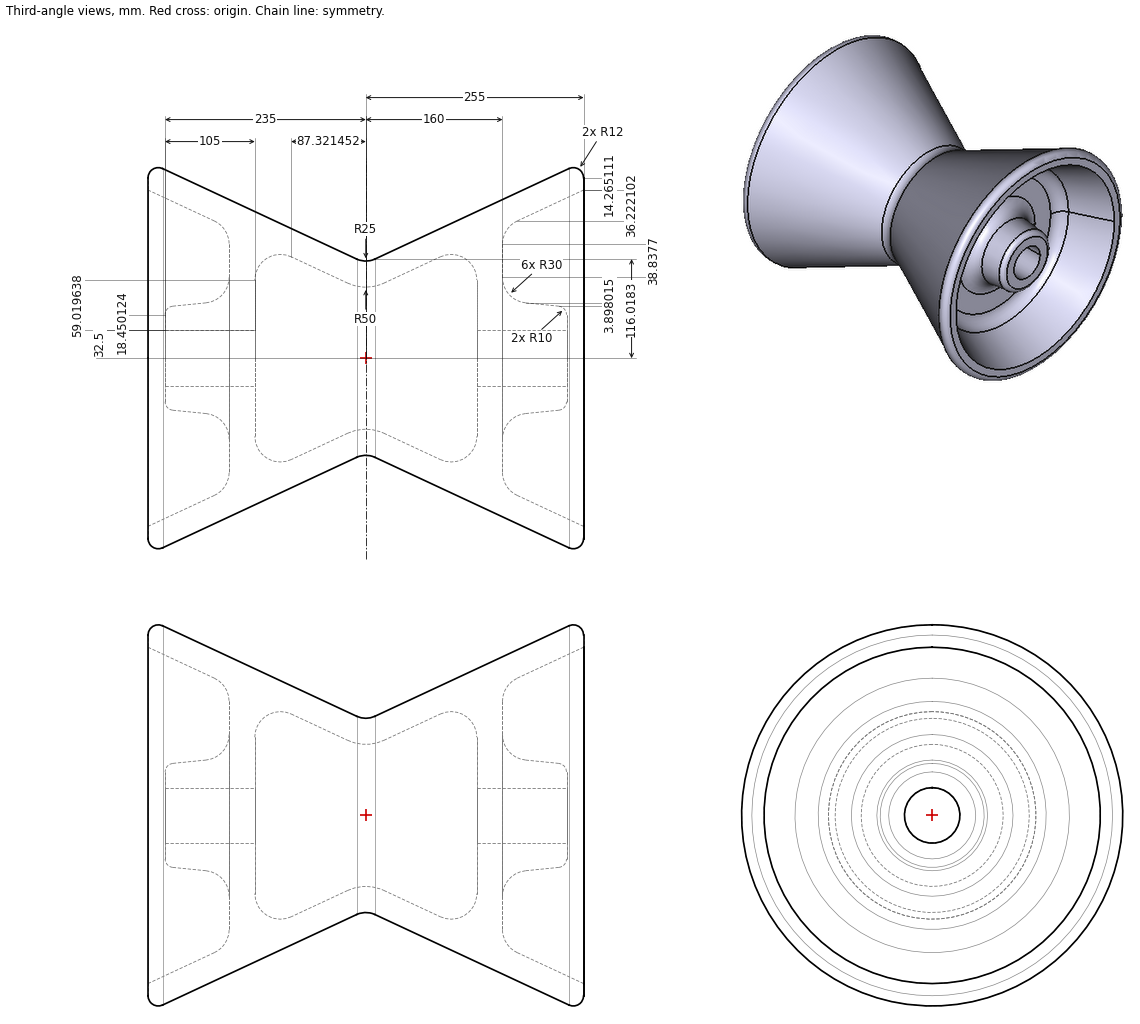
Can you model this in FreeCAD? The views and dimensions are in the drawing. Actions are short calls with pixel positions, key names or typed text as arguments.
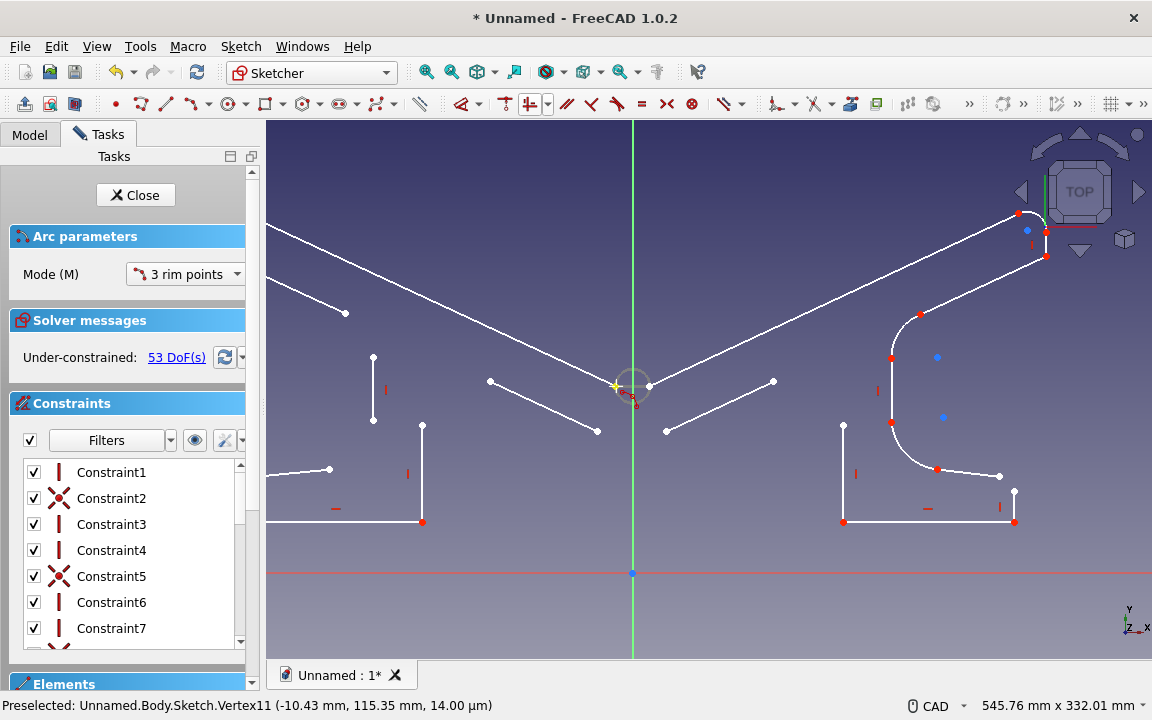
scroll(629, 389, up, 8)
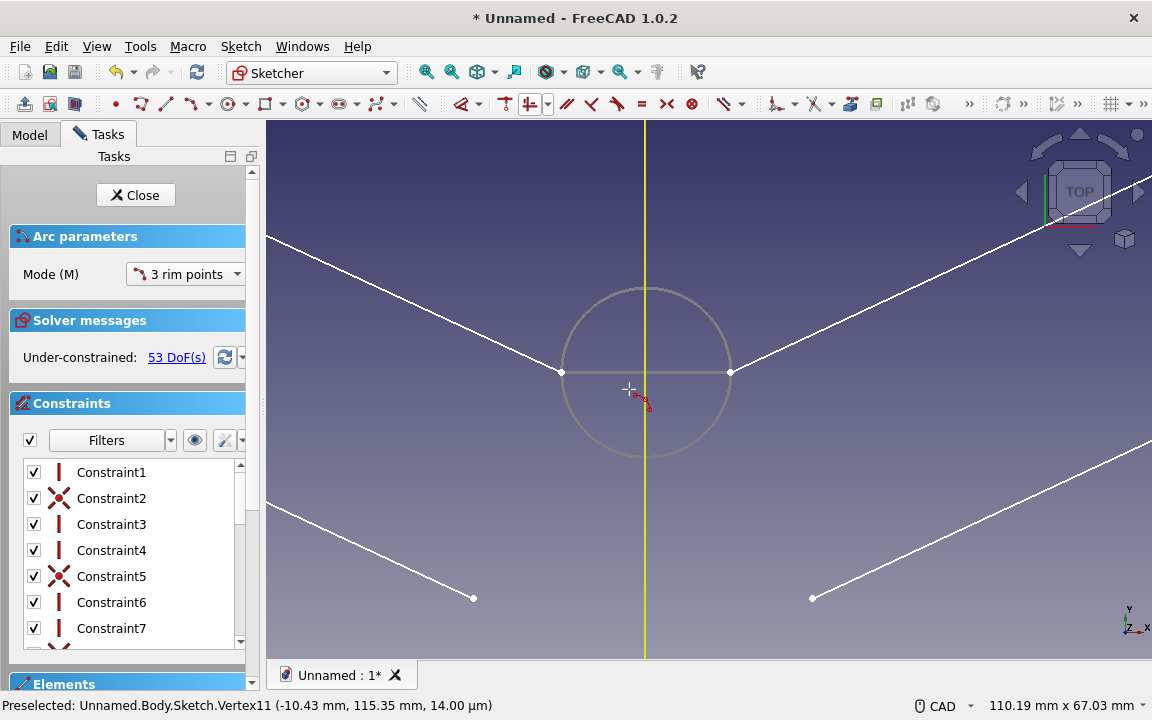
click(628, 385)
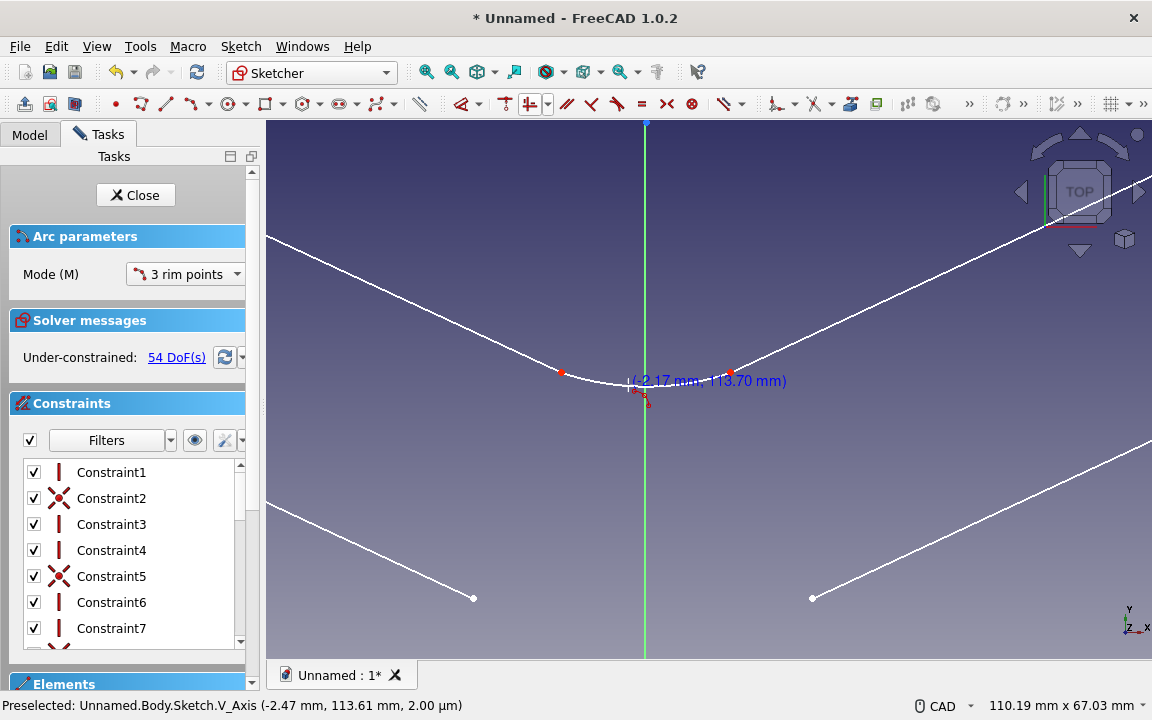
scroll(640, 387, down, 11)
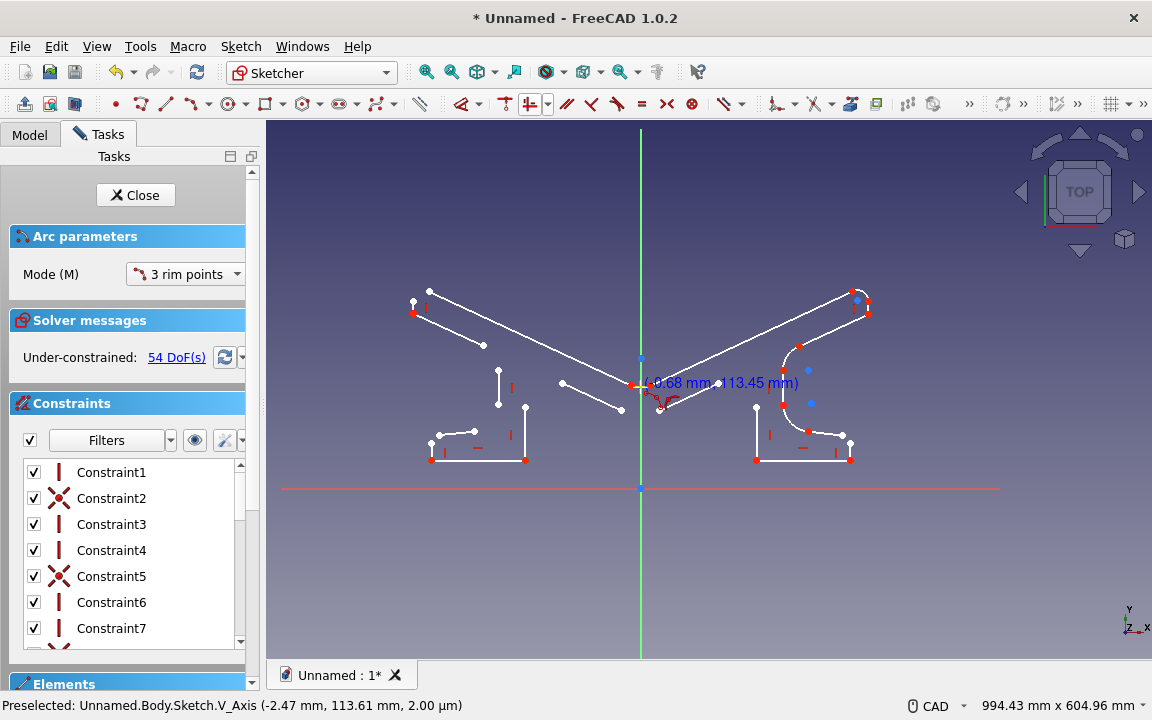
click(429, 292)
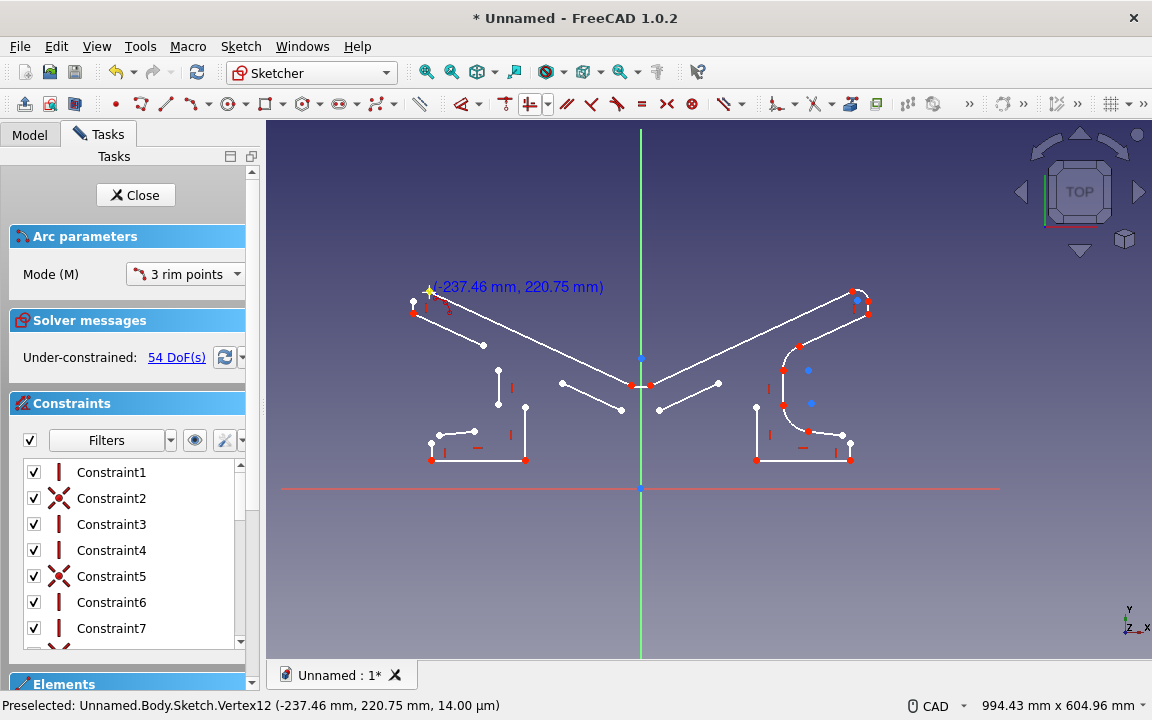
scroll(414, 300, up, 5)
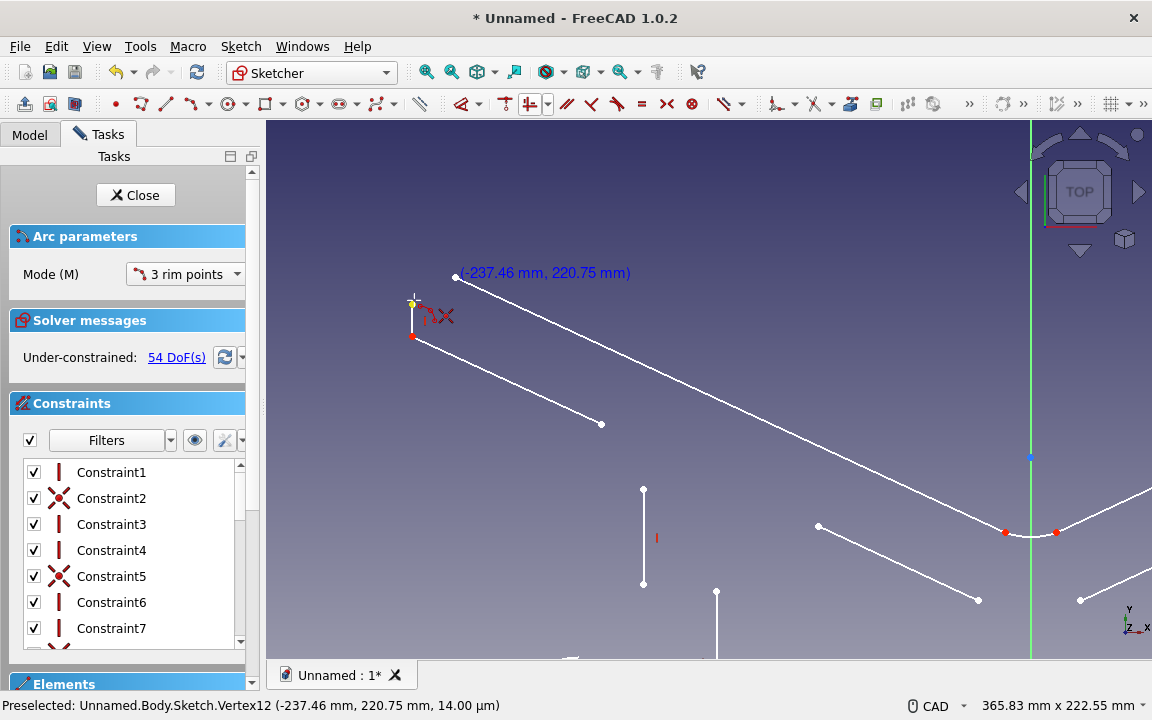
click(412, 305)
click(427, 276)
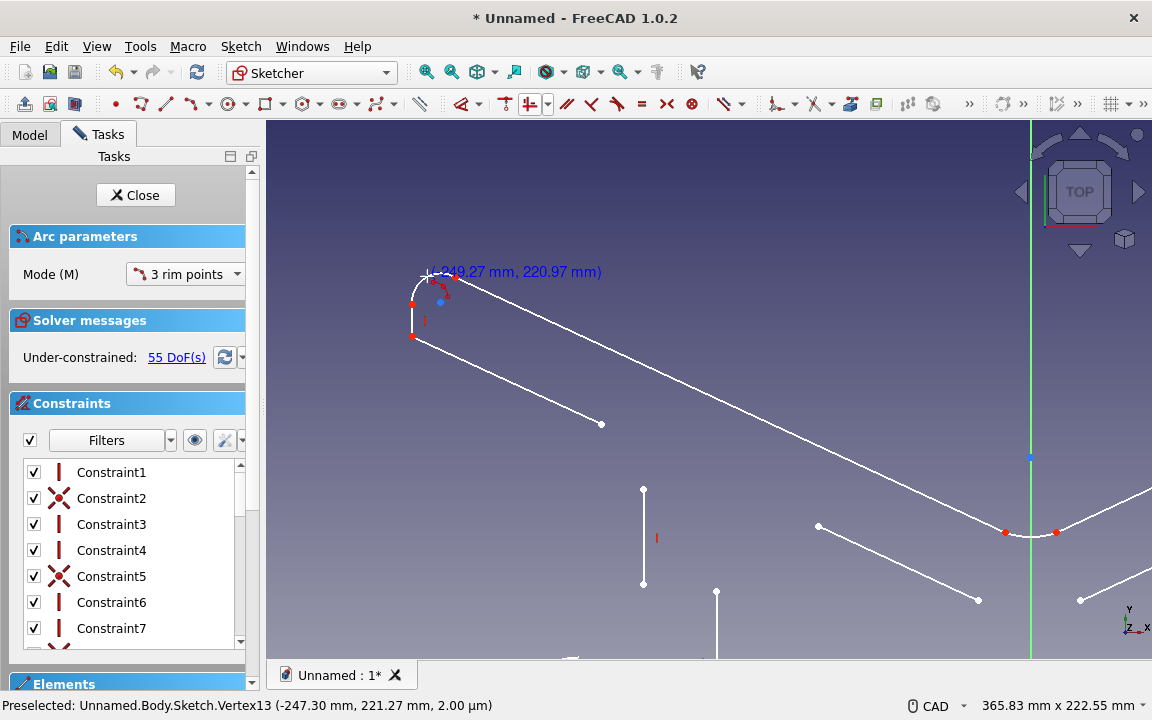
click(602, 424)
click(644, 490)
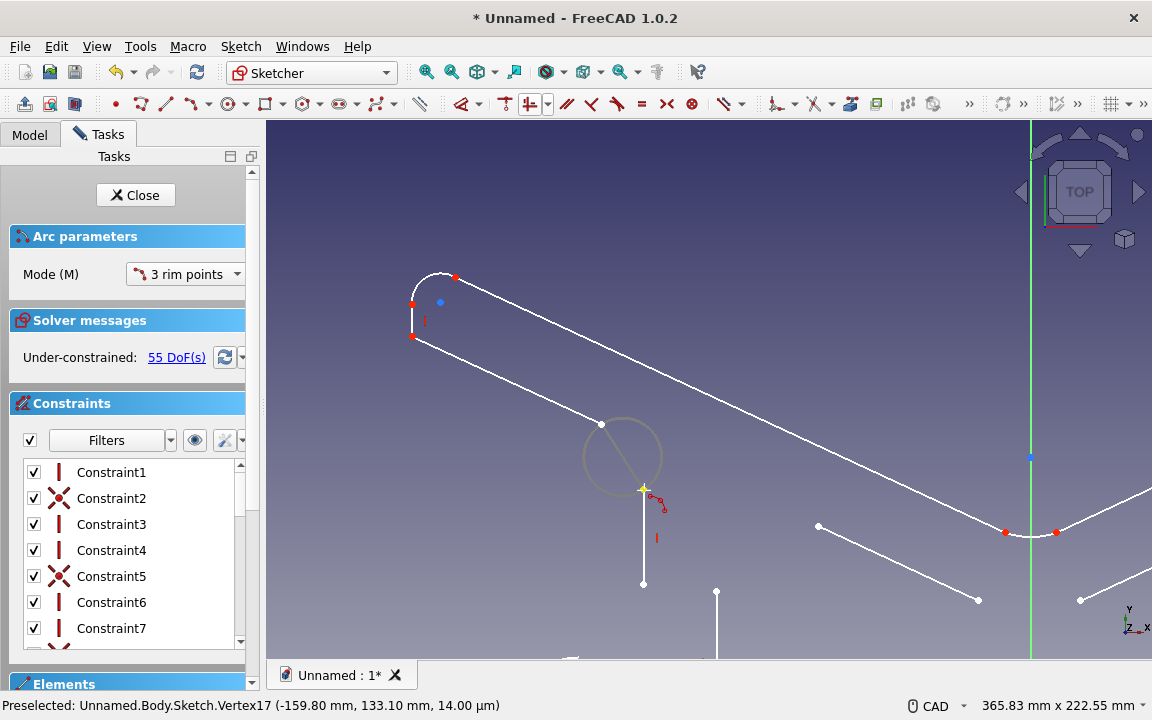
scroll(632, 450, up, 2)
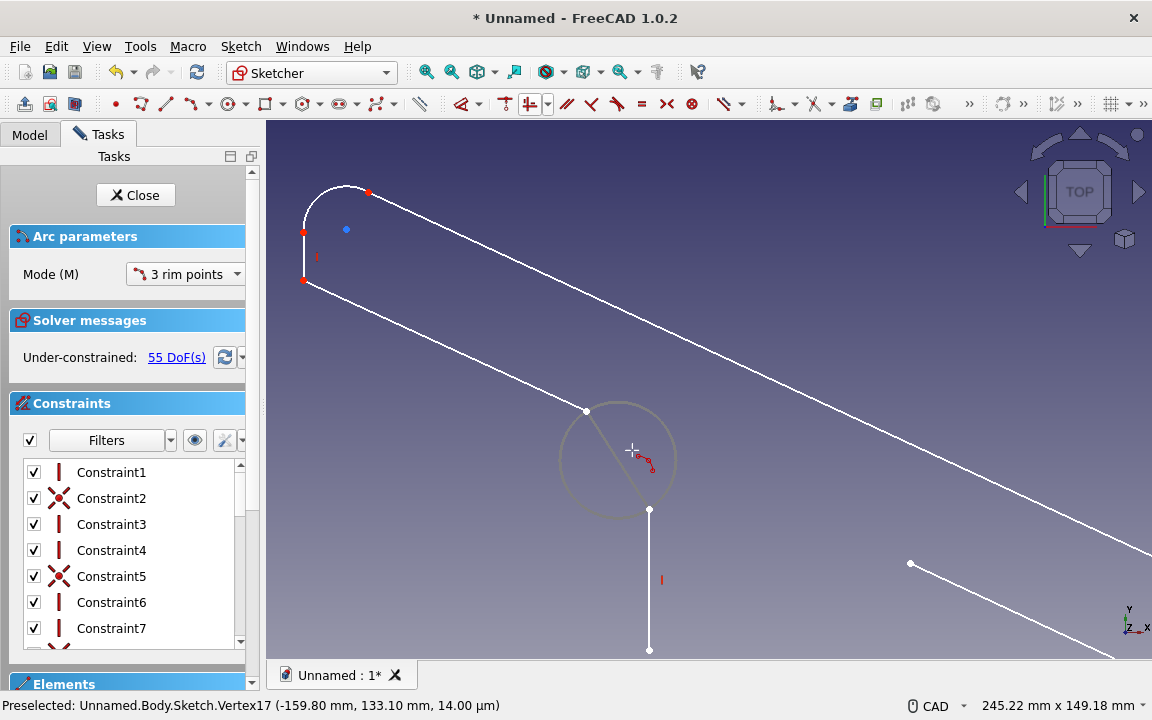
click(632, 449)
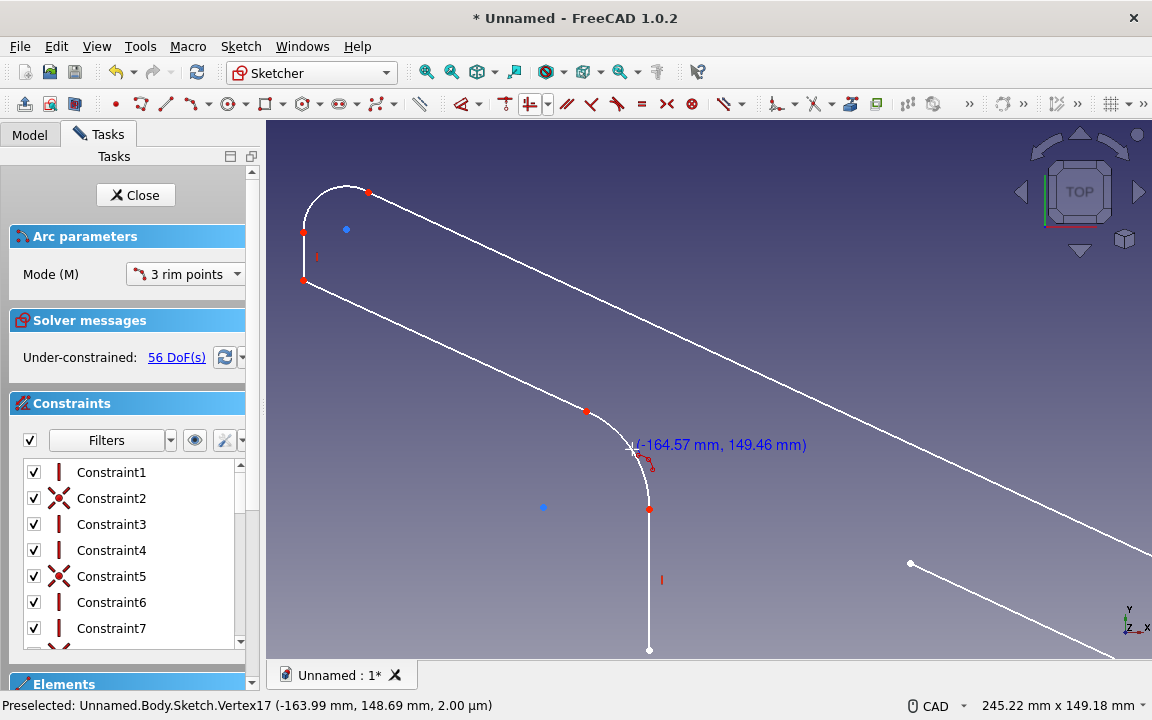
scroll(449, 324, down, 7)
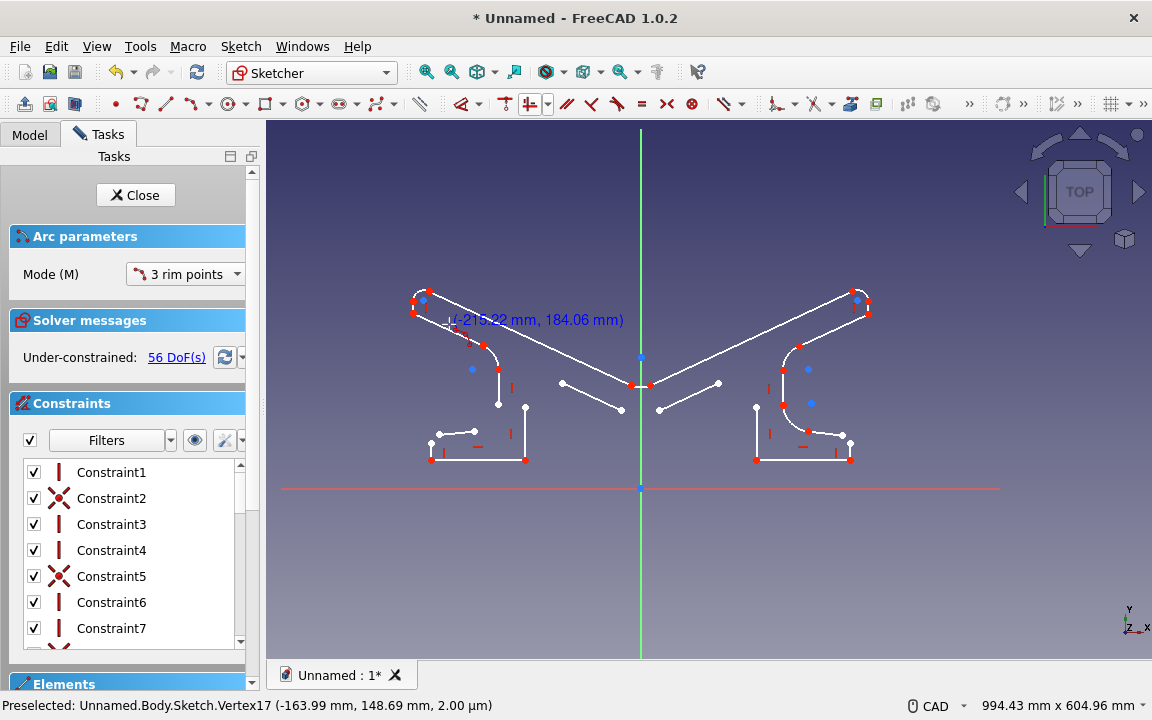
click(499, 405)
click(474, 432)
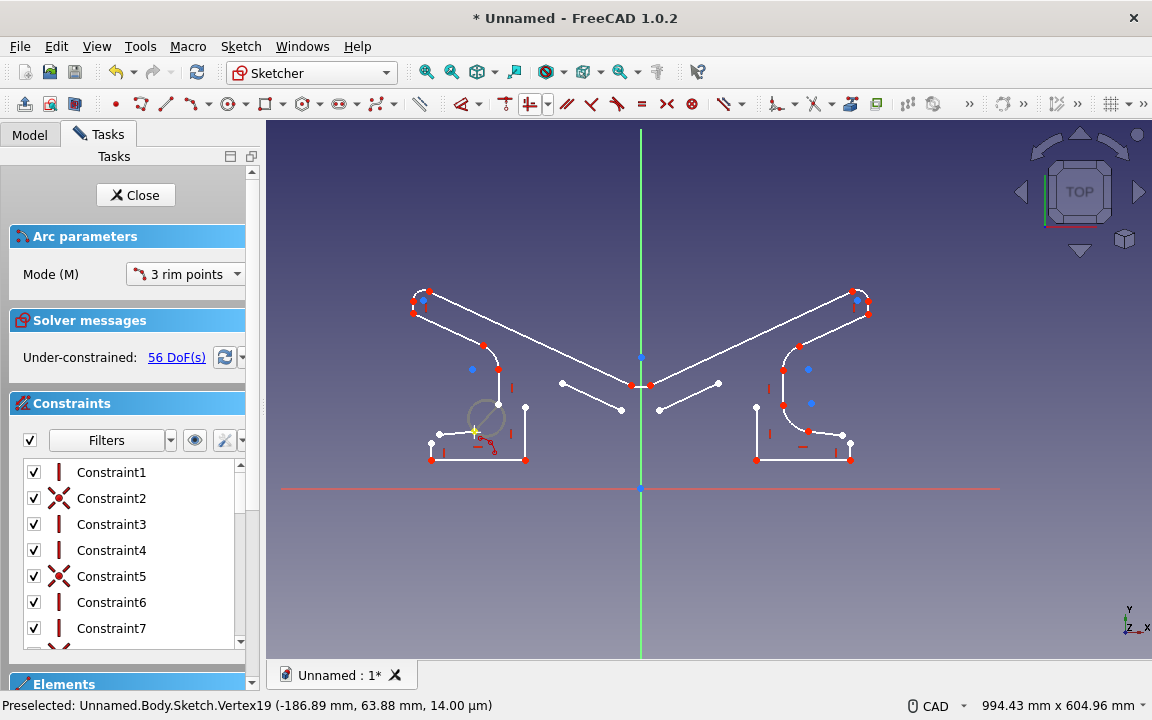
scroll(491, 422, up, 5)